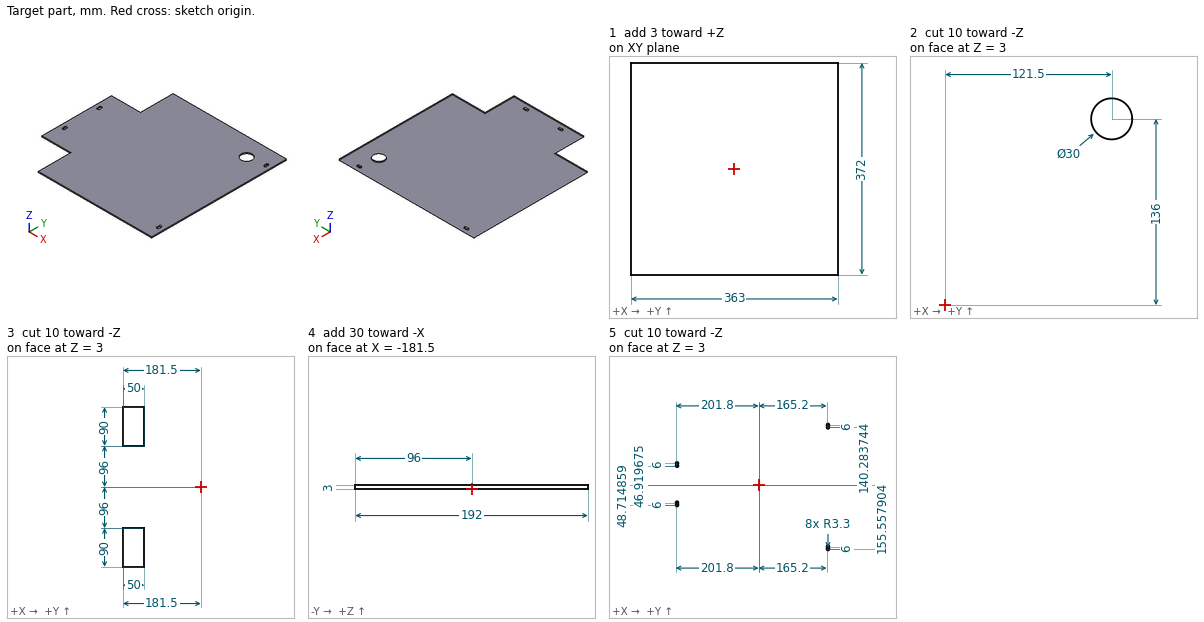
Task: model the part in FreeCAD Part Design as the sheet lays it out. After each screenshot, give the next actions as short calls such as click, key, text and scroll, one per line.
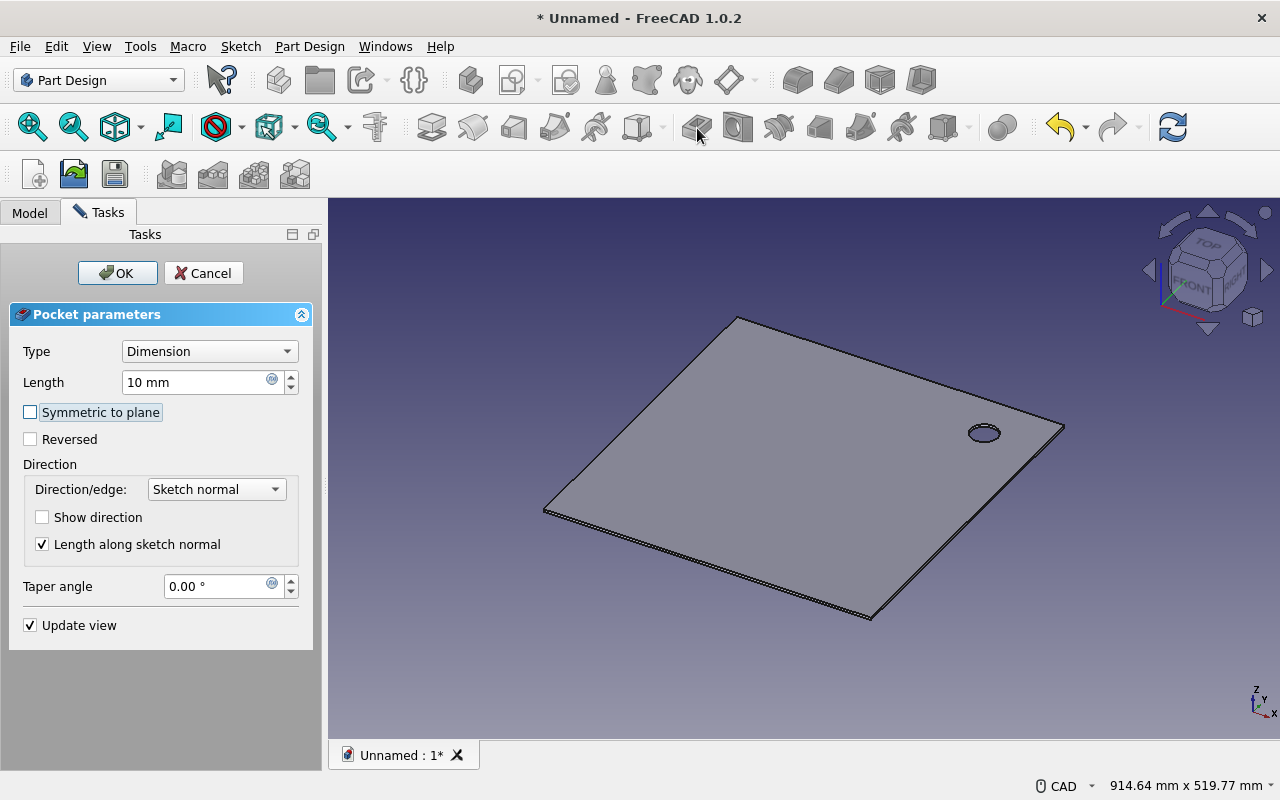
click(118, 273)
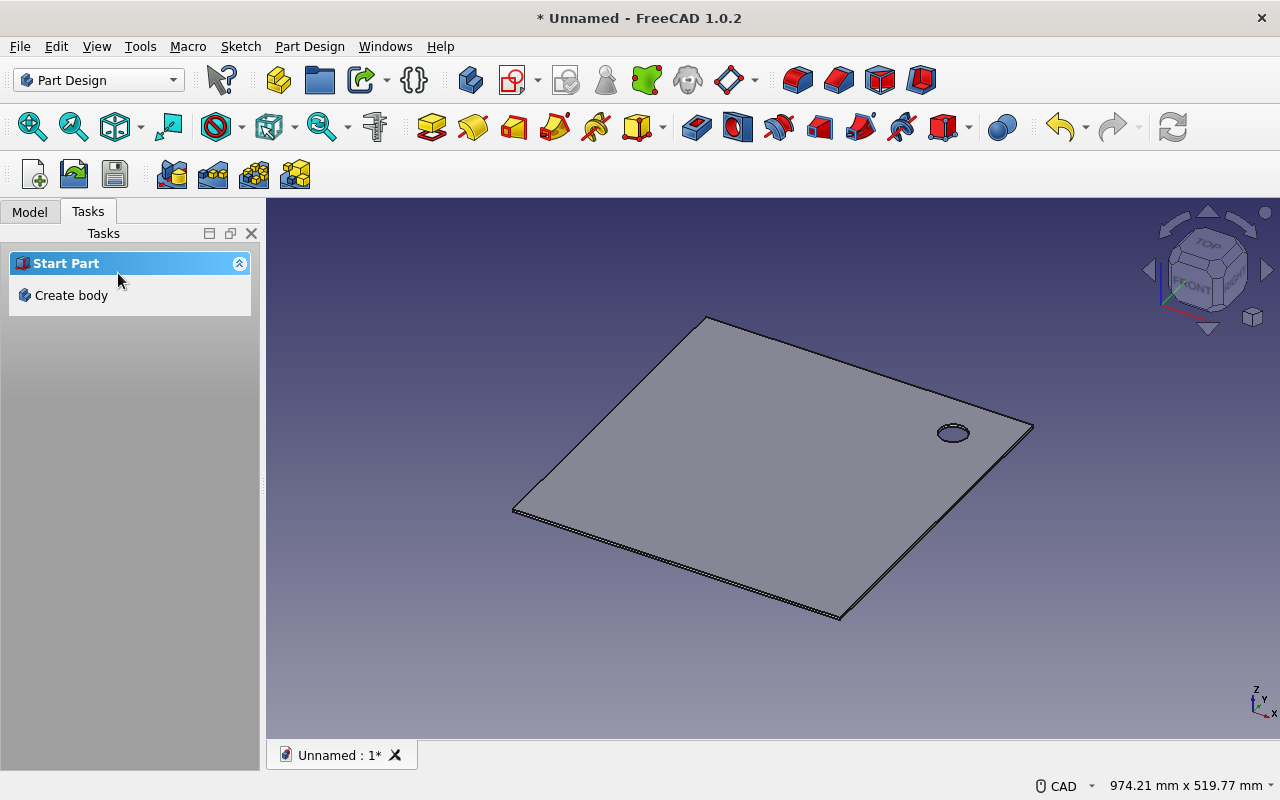
click(773, 466)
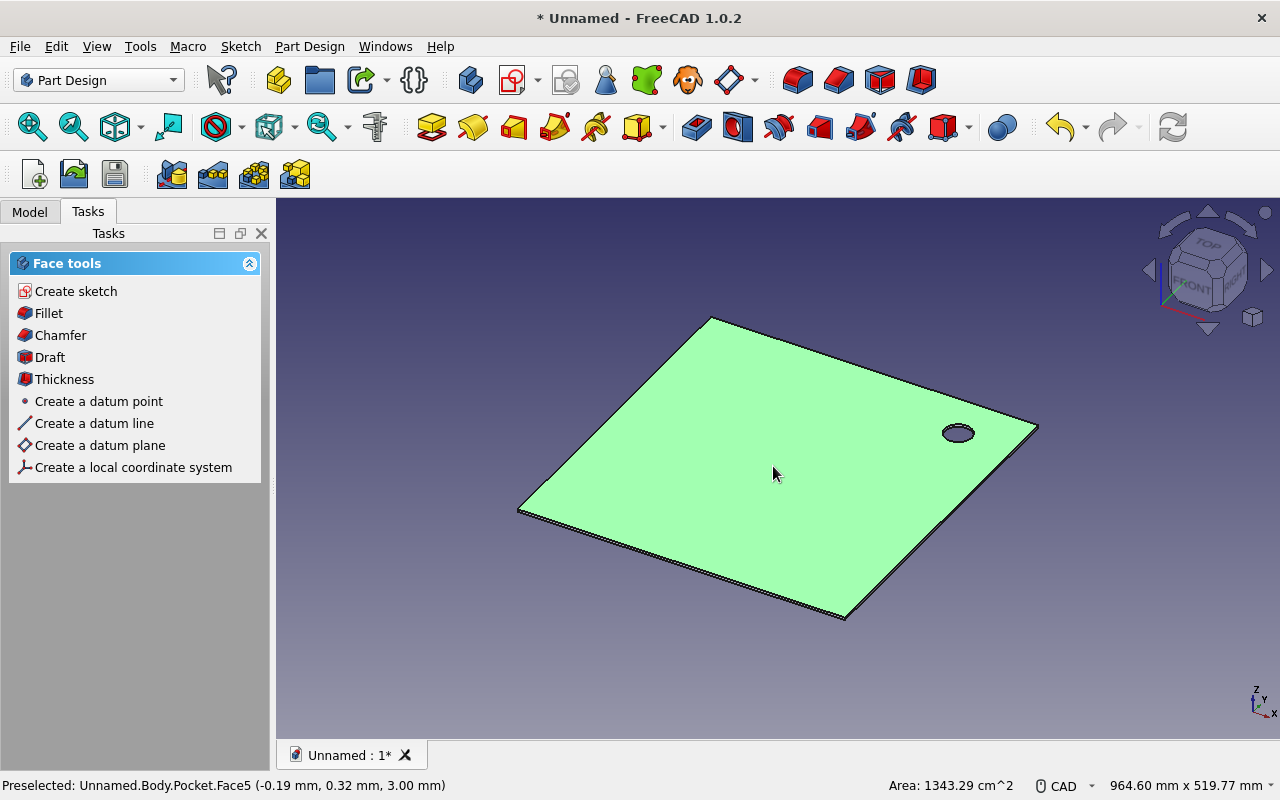
click(512, 80)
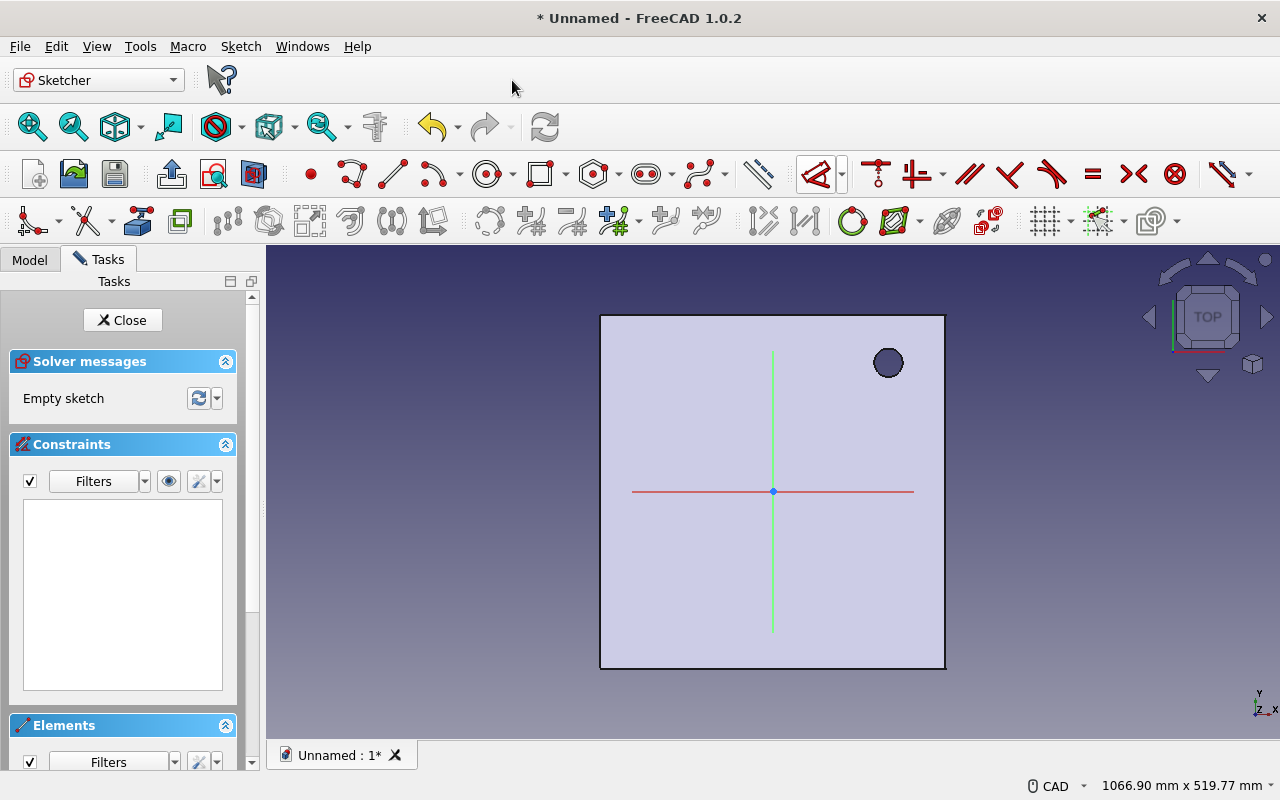
click(540, 174)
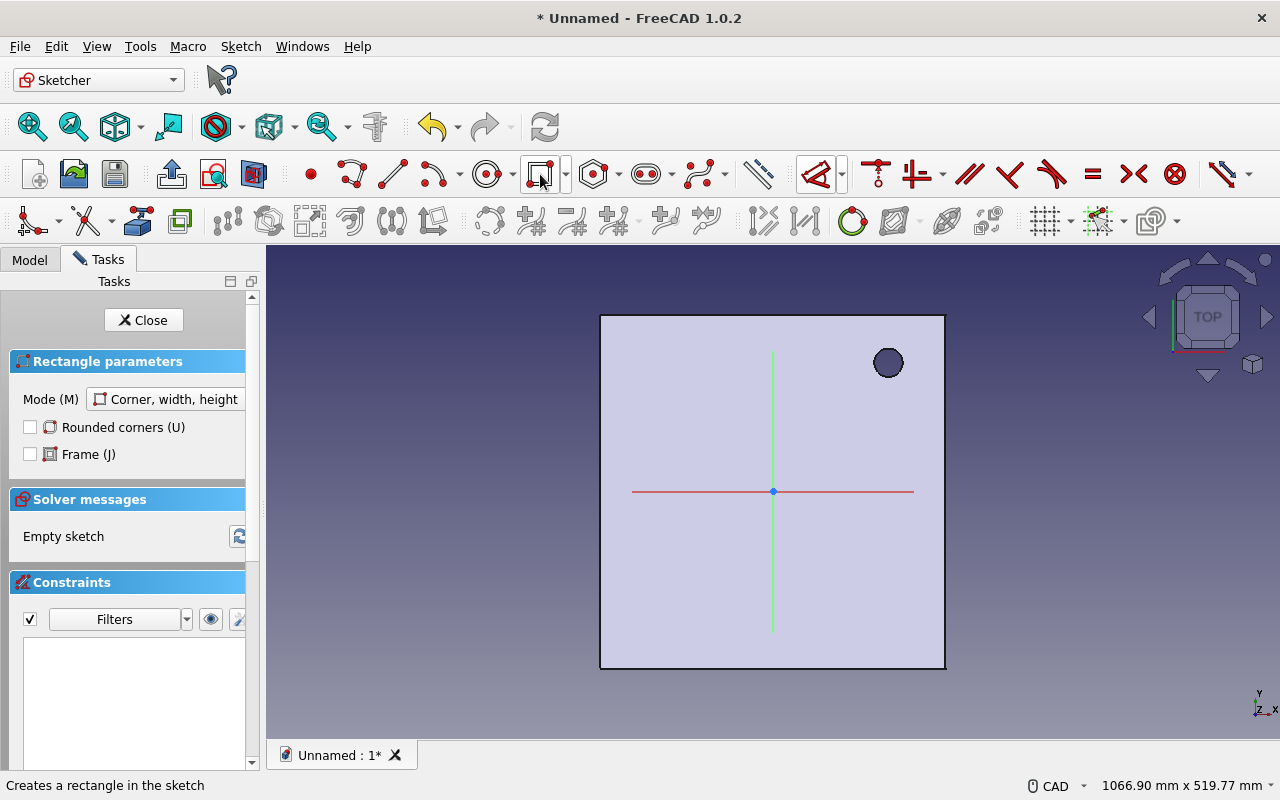
click(600, 583)
move(648, 669)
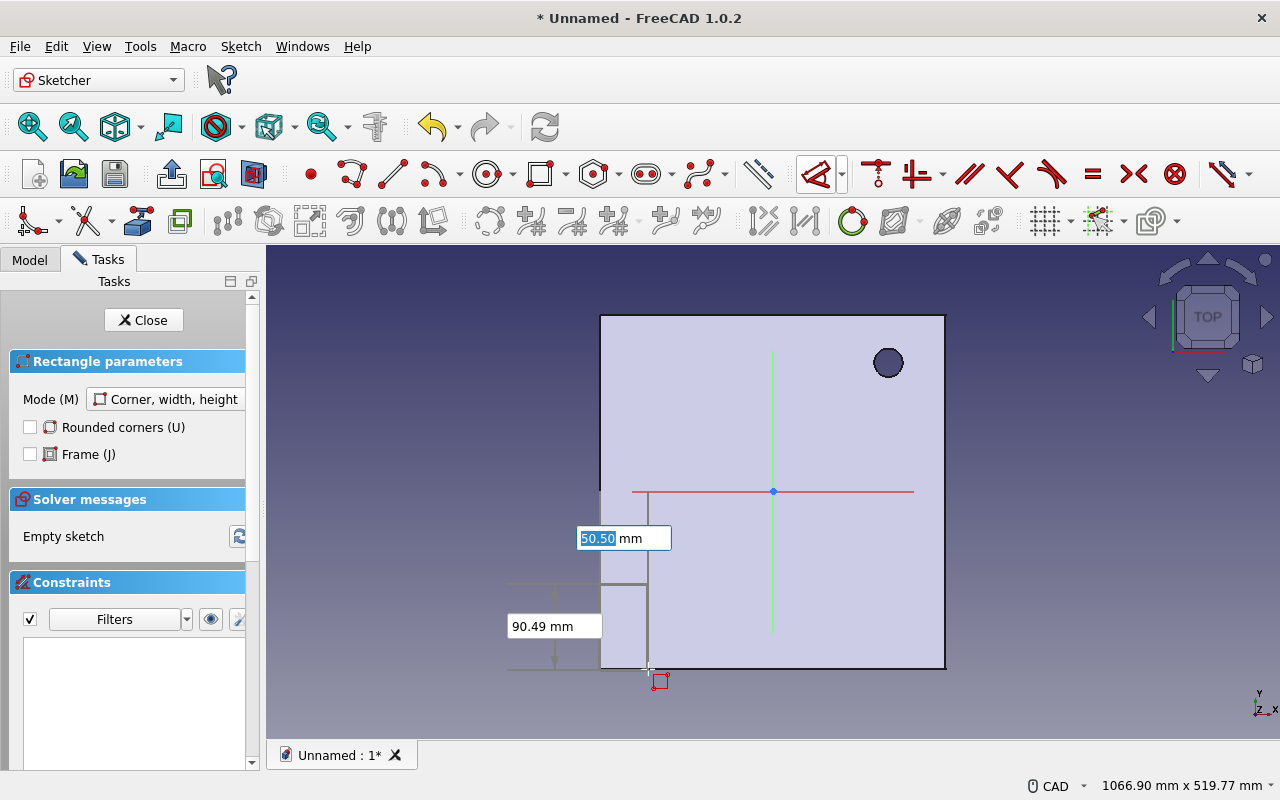
text(50)
key(Tab)
text(90)
key(Return)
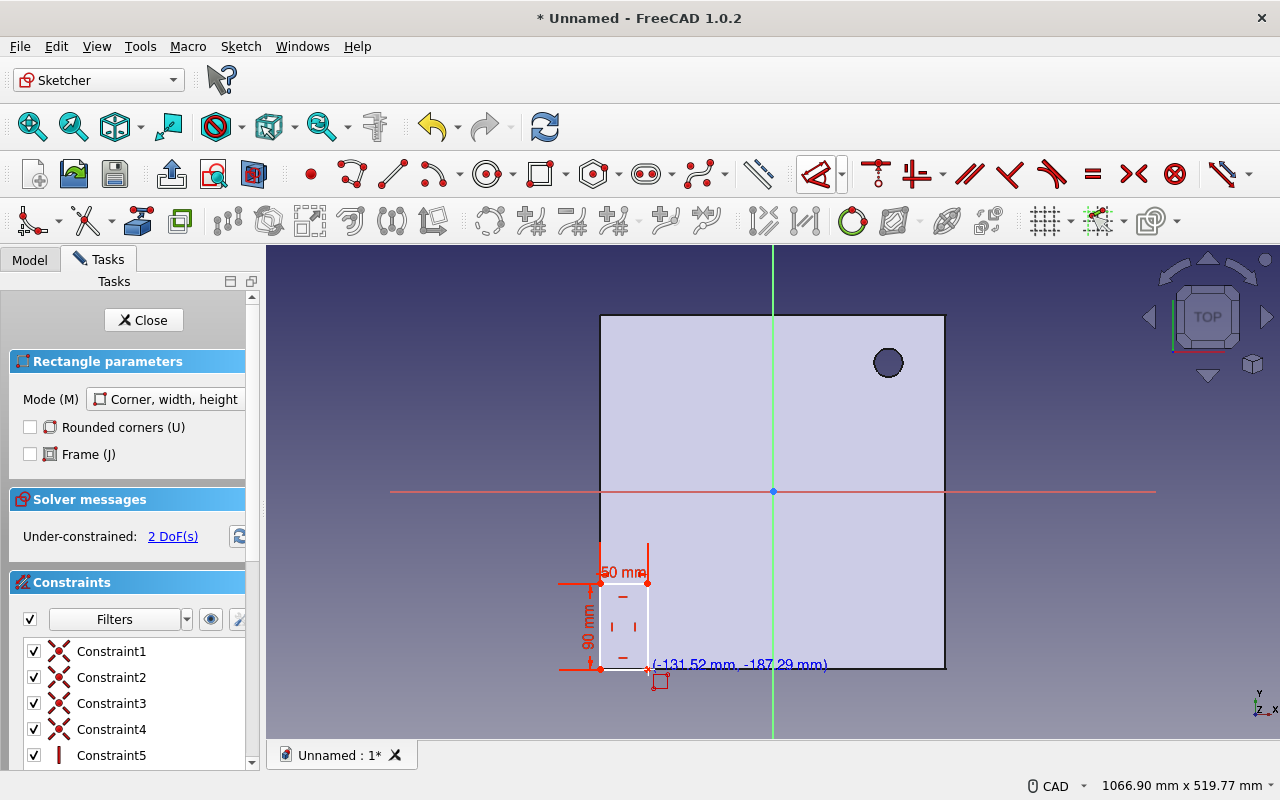
click(600, 315)
move(648, 401)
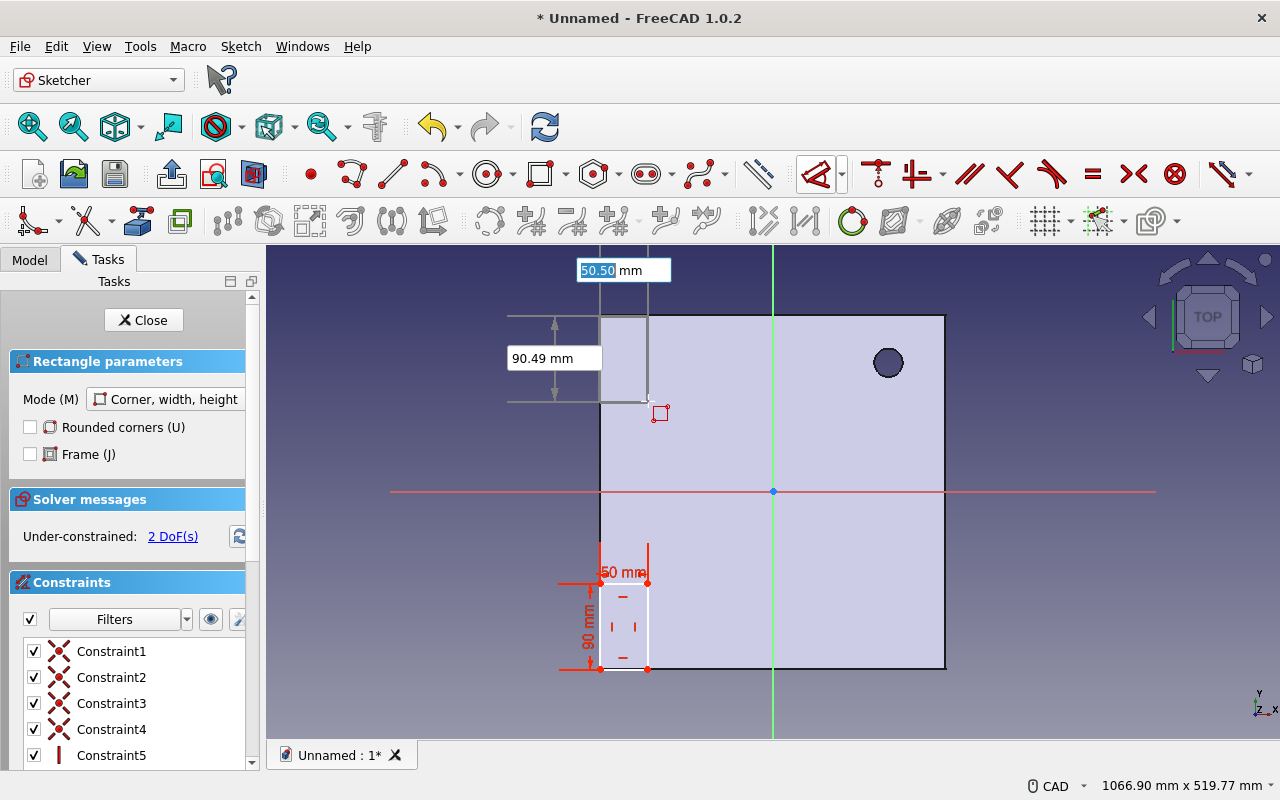
text(50)
key(Tab)
text(90)
key(Return)
key(Escape)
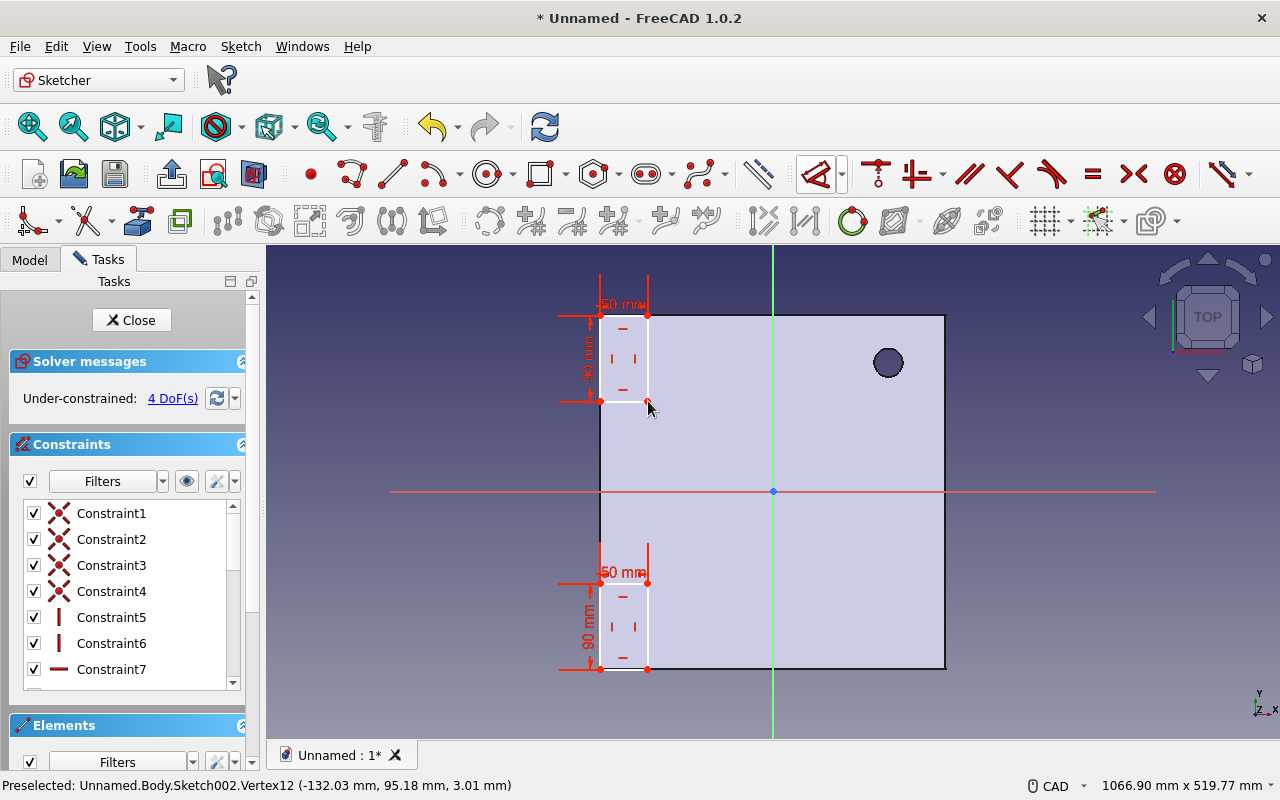
click(600, 584)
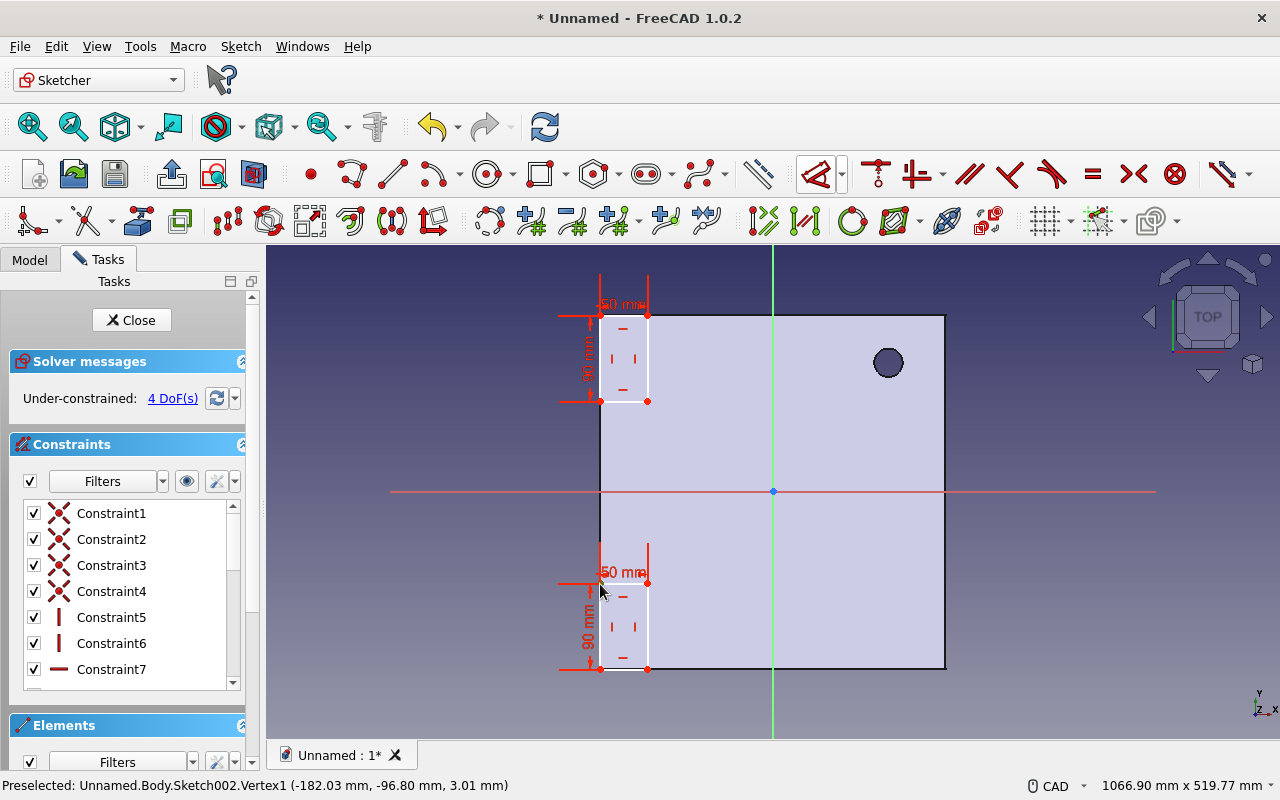
key(i)